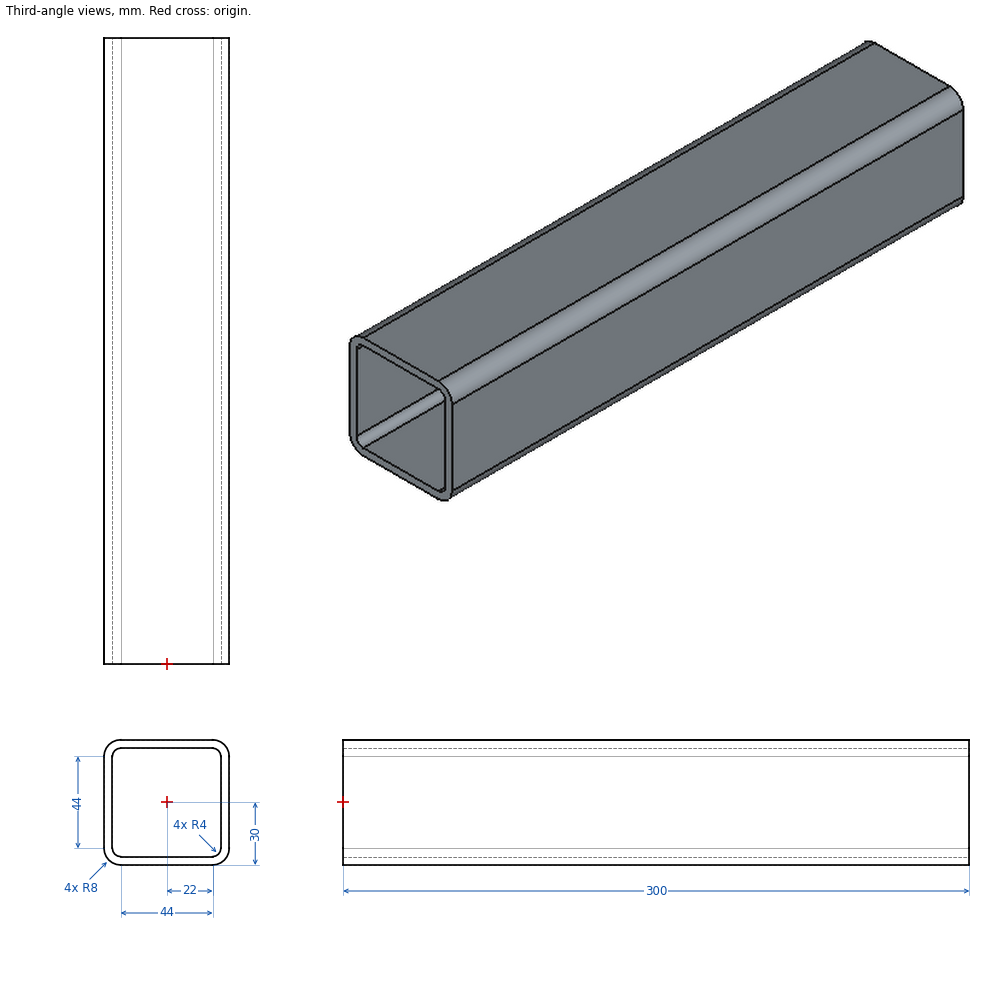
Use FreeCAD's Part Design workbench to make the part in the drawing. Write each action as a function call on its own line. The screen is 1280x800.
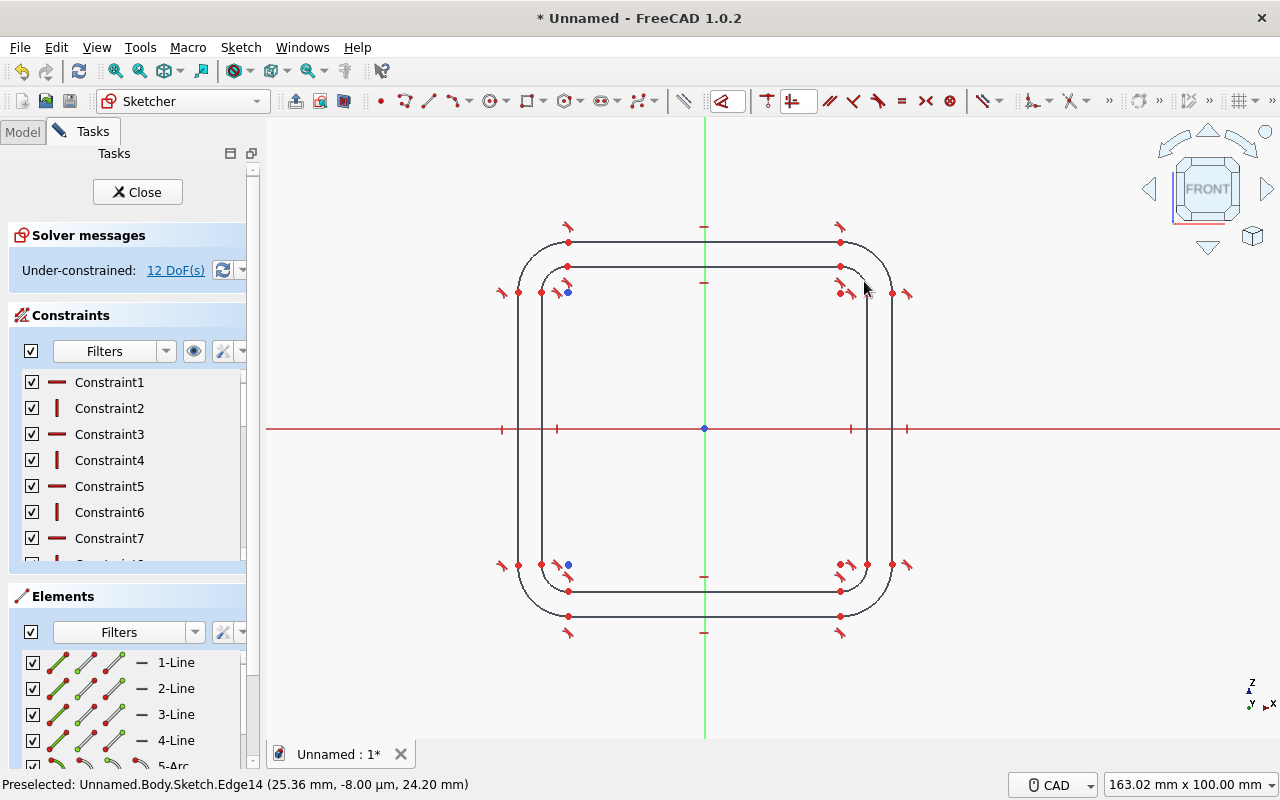
click(546, 248)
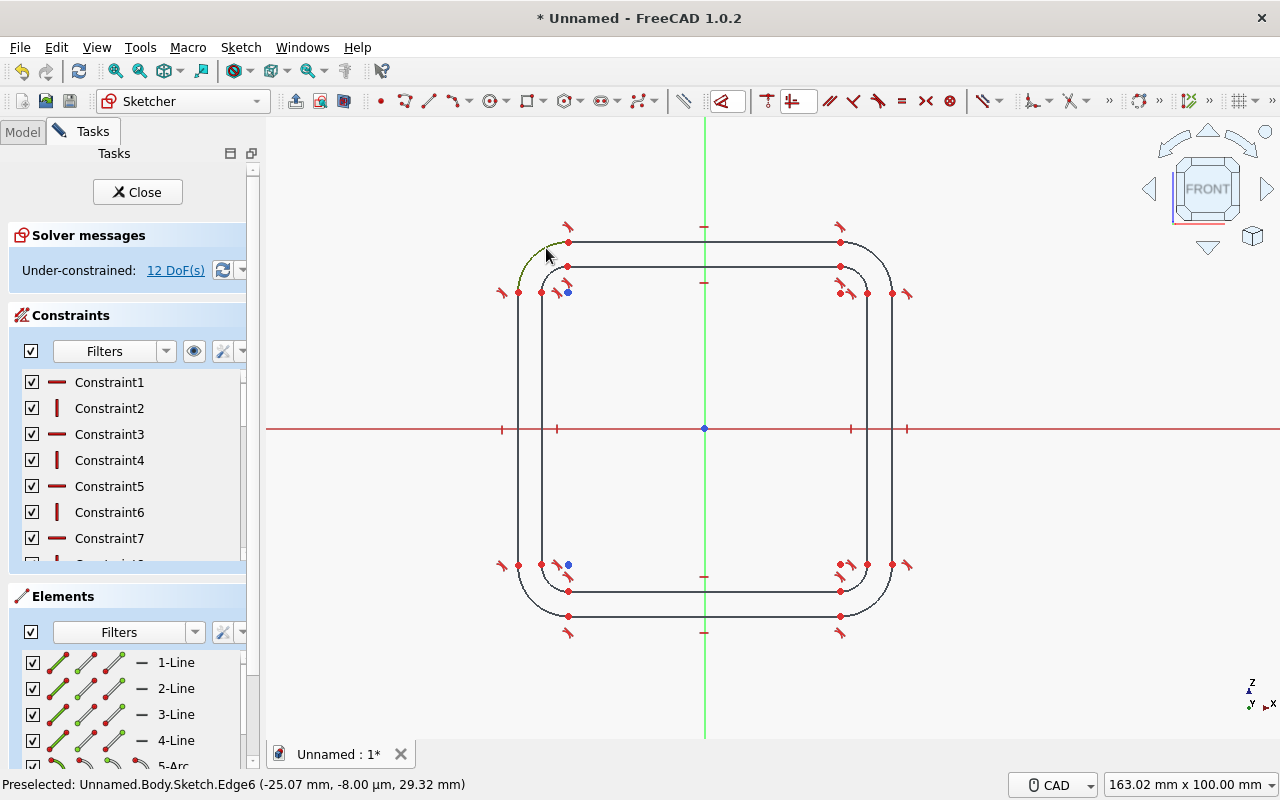
click(556, 270)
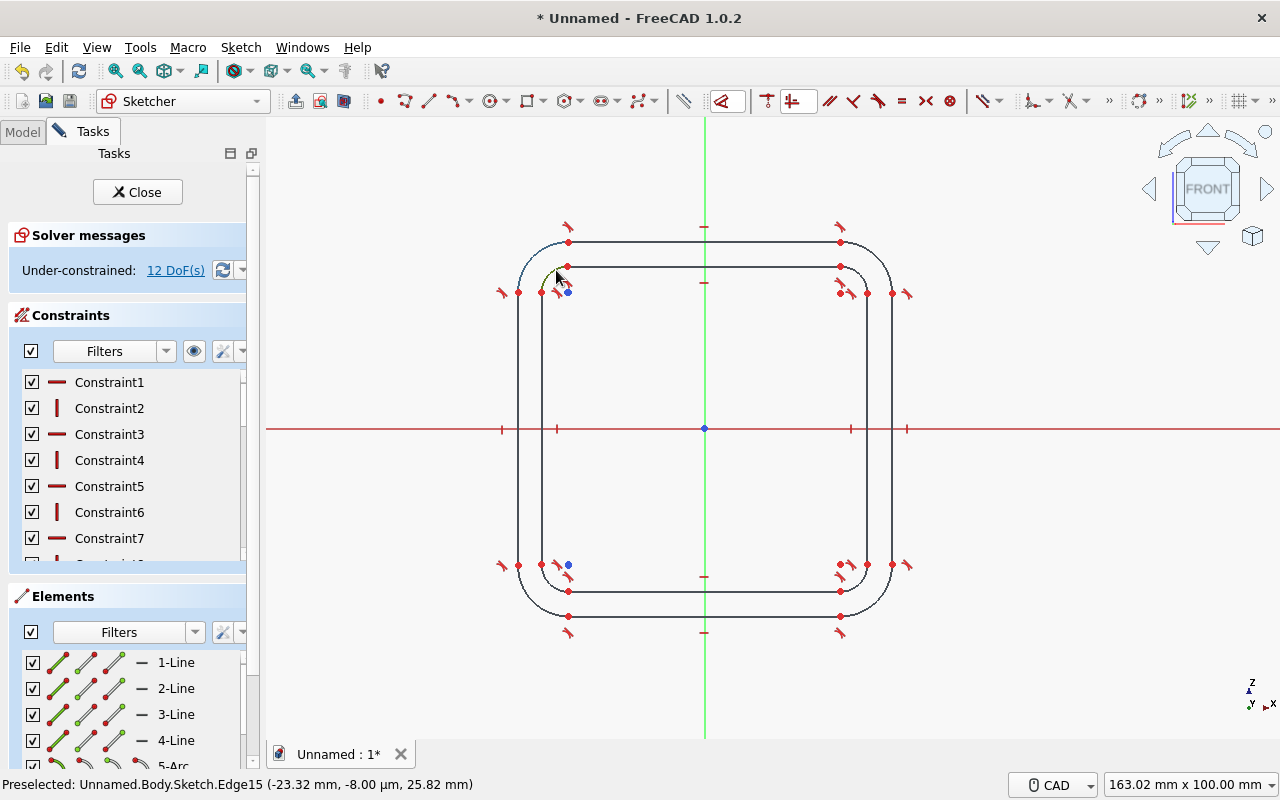
key(c)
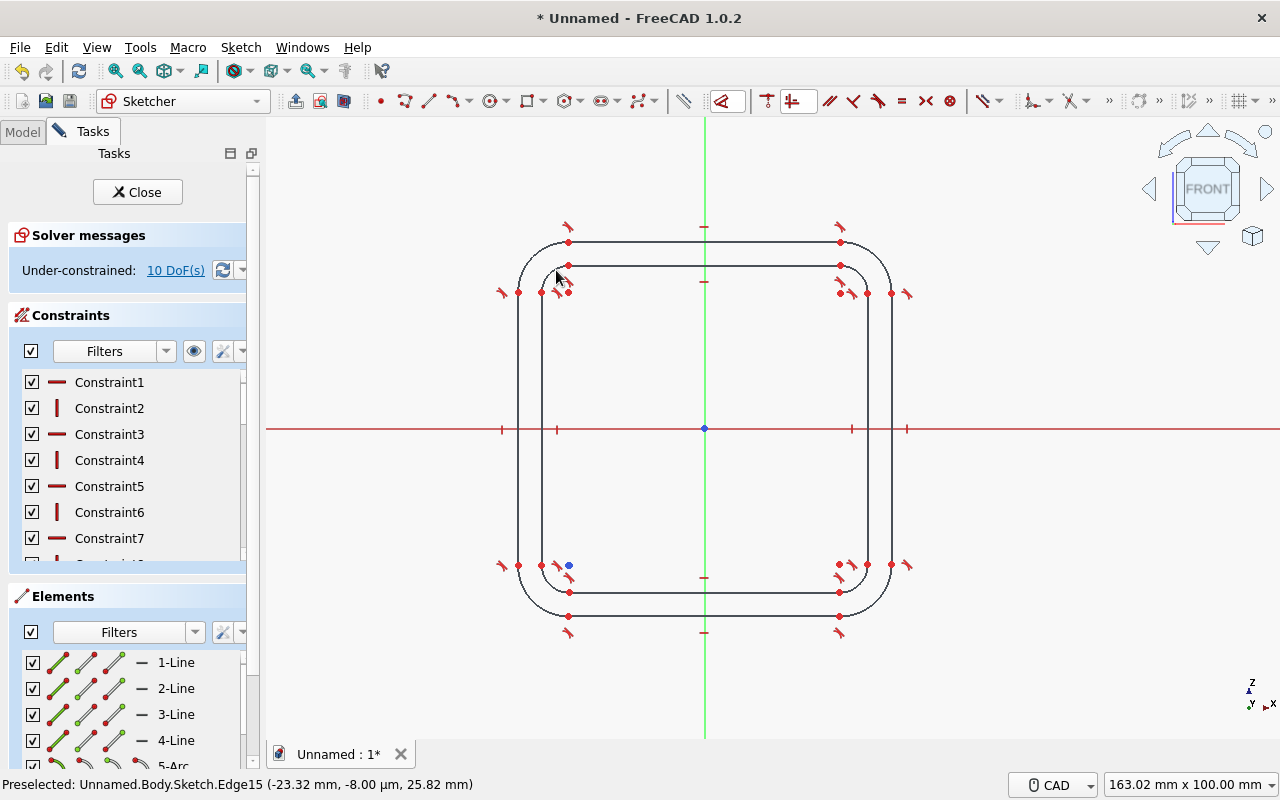
click(524, 589)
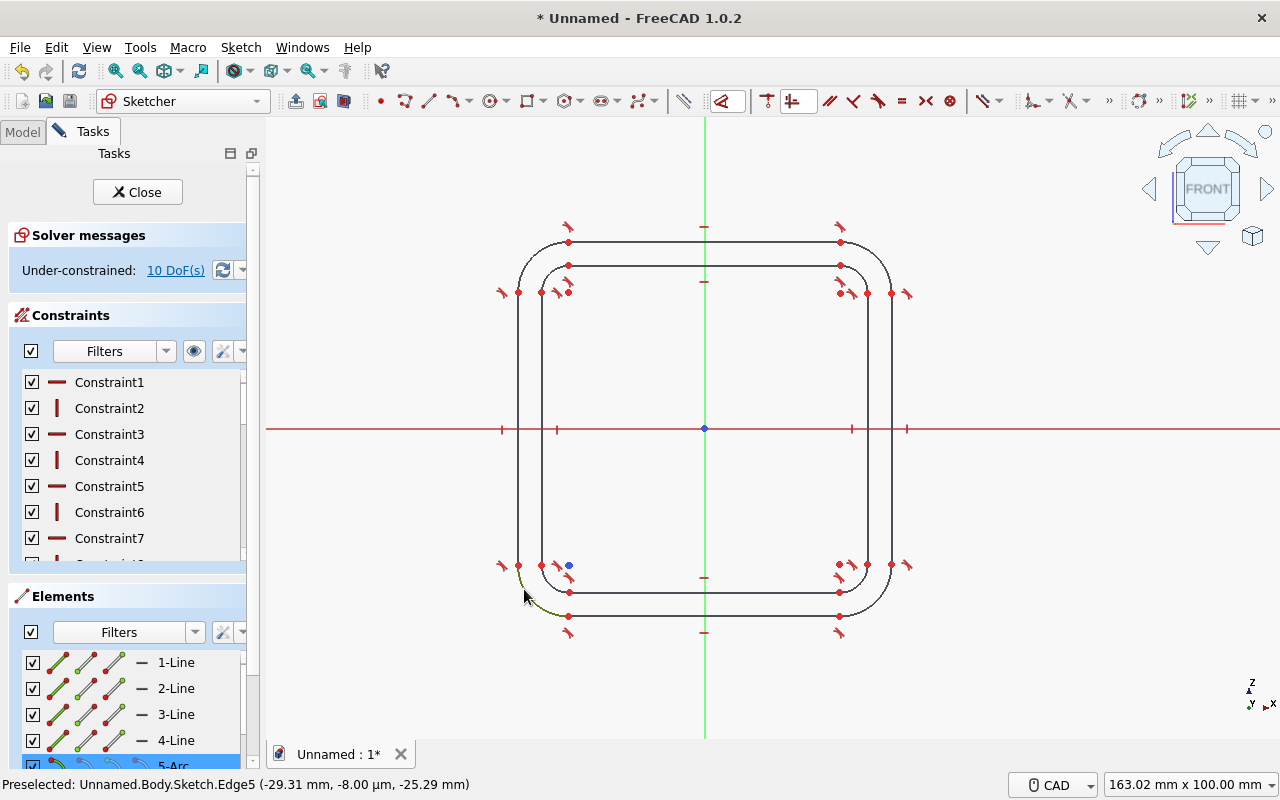
click(546, 248)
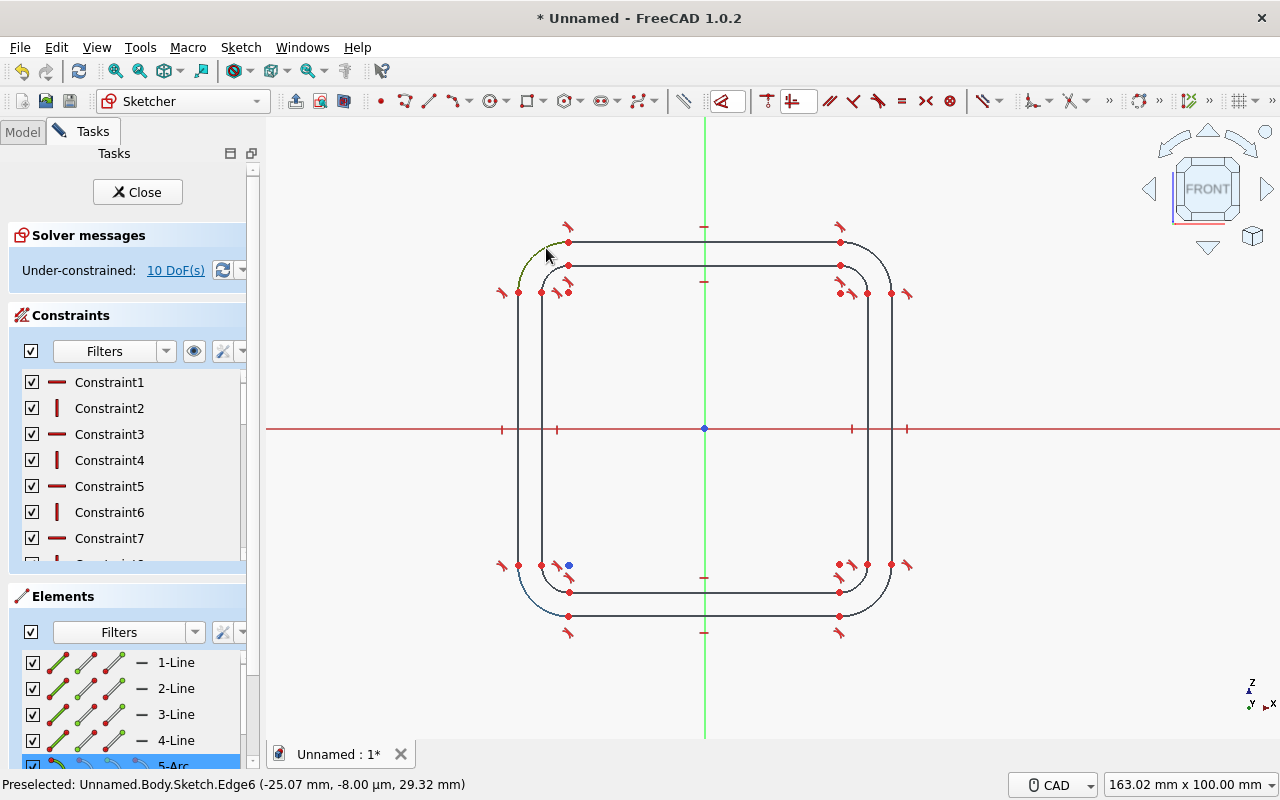
click(886, 270)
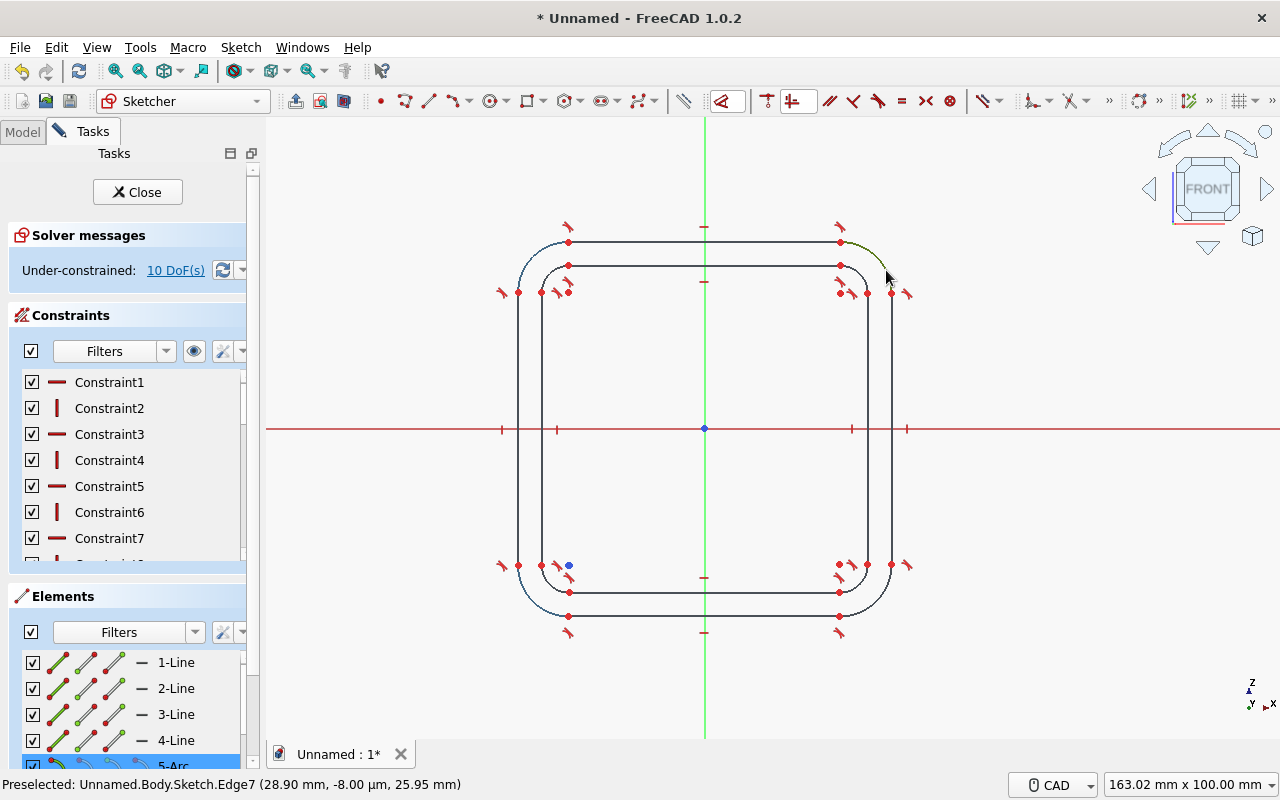
click(863, 611)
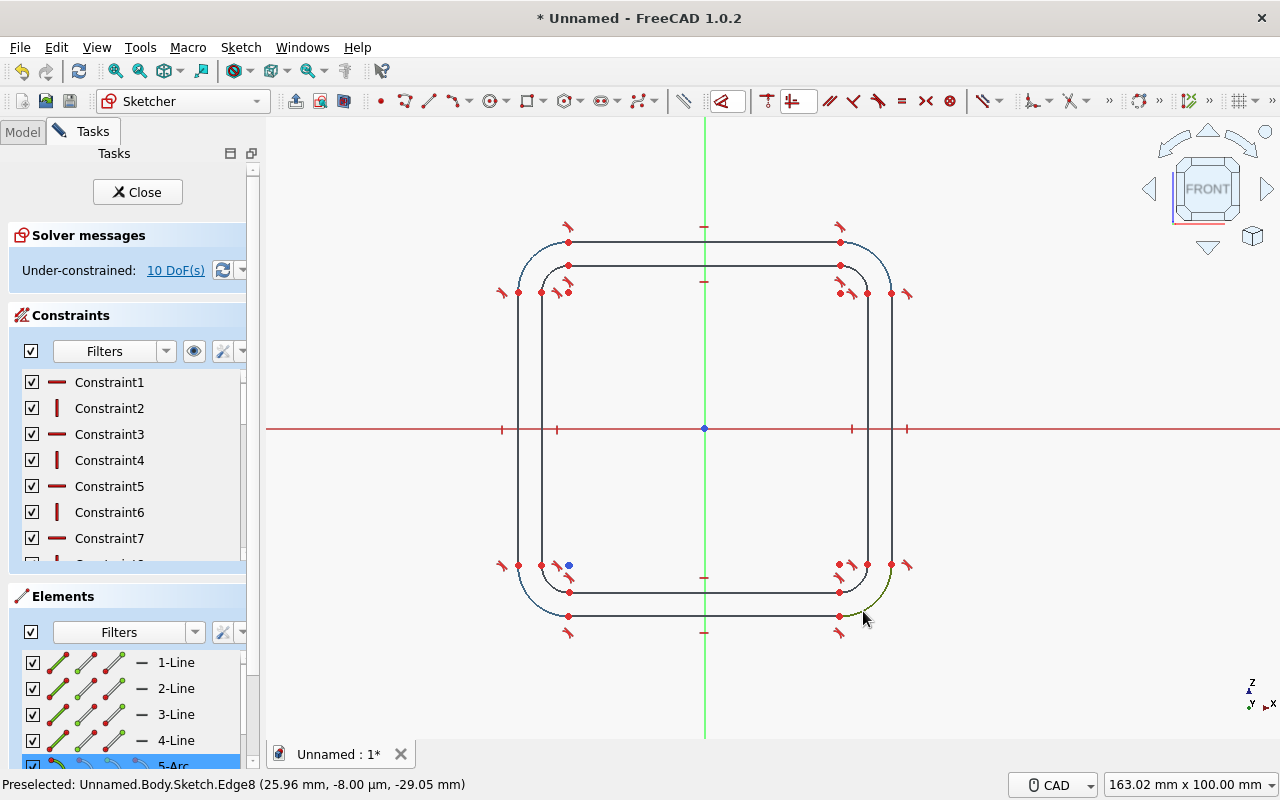
click(902, 102)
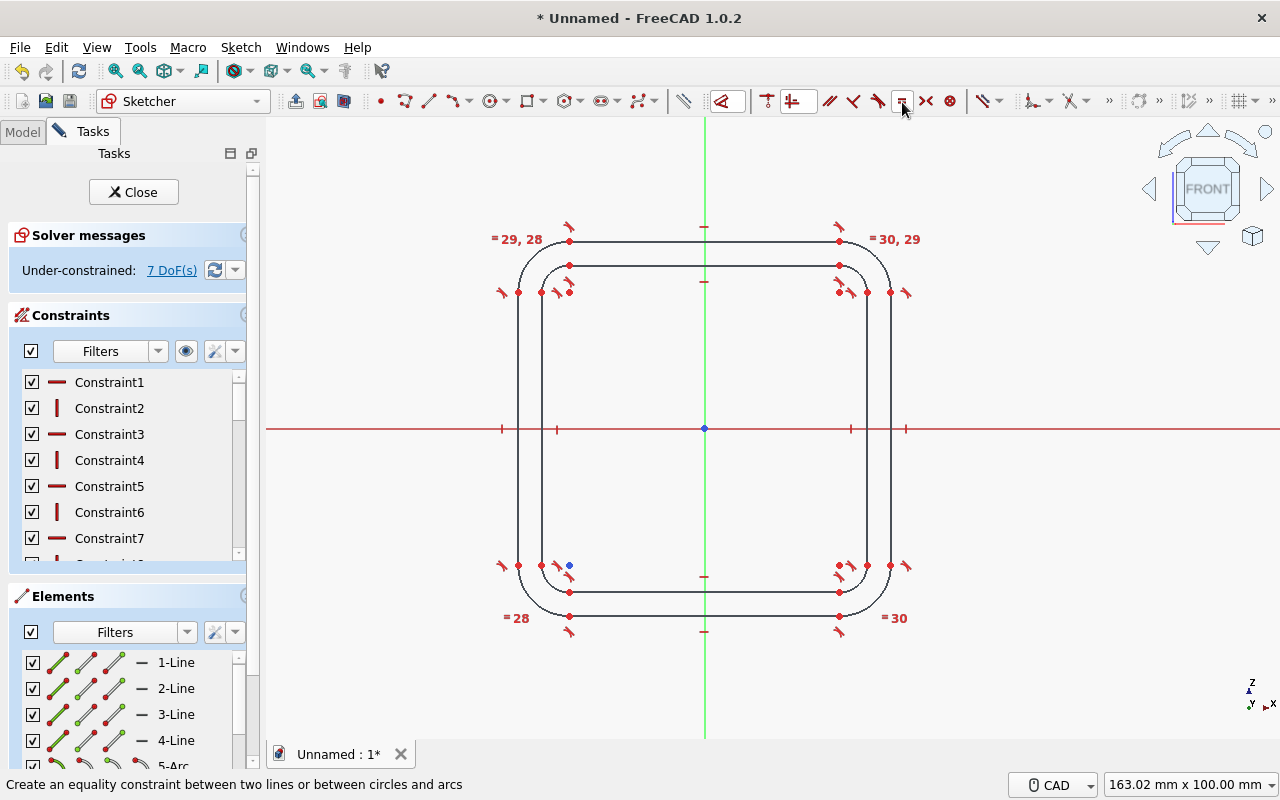
click(852, 589)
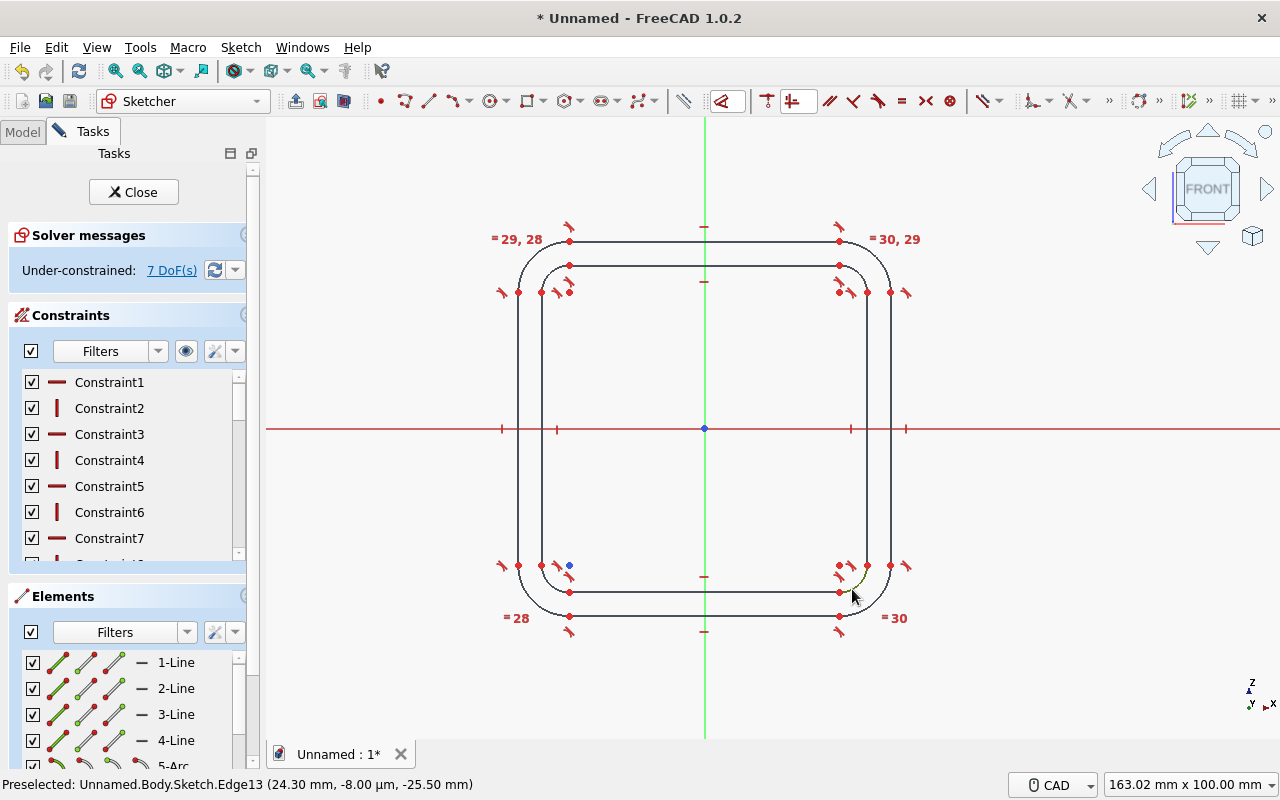
click(545, 578)